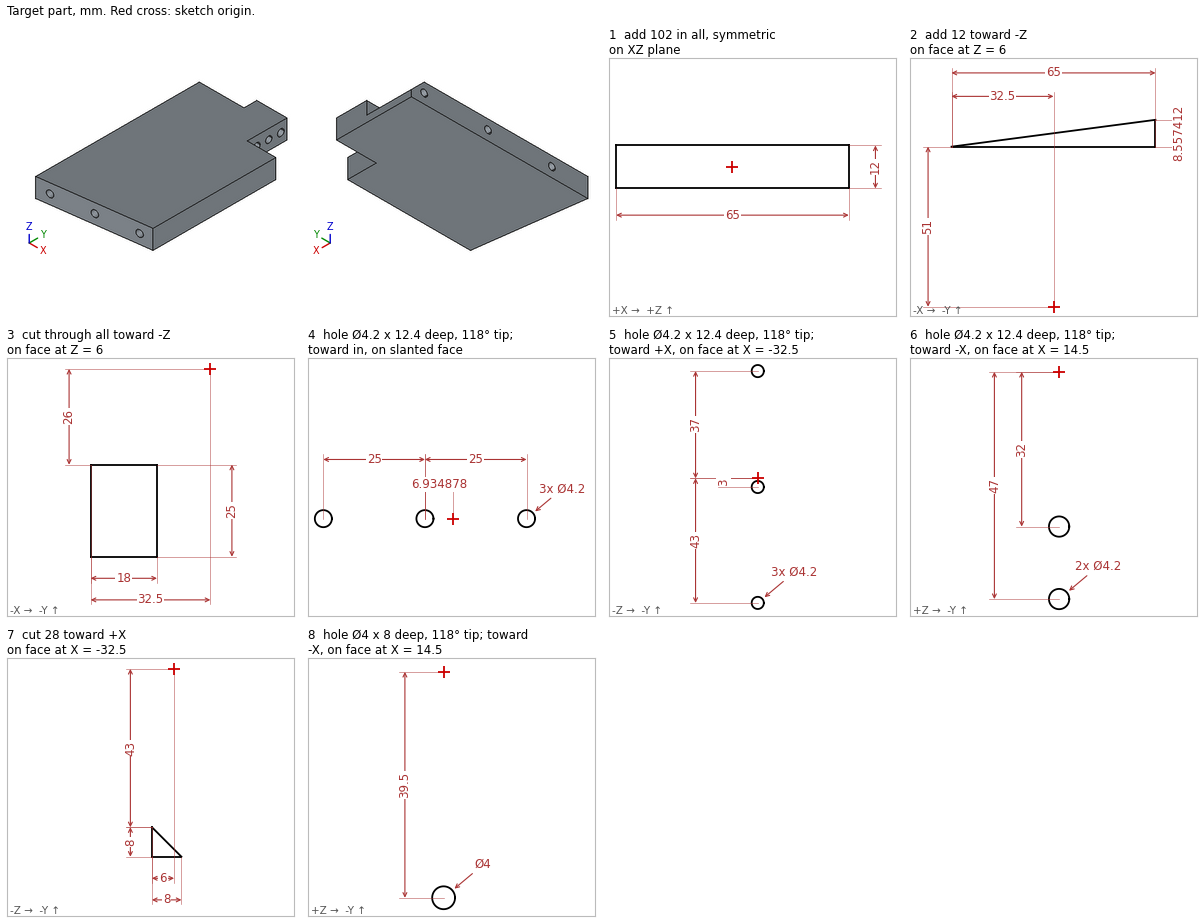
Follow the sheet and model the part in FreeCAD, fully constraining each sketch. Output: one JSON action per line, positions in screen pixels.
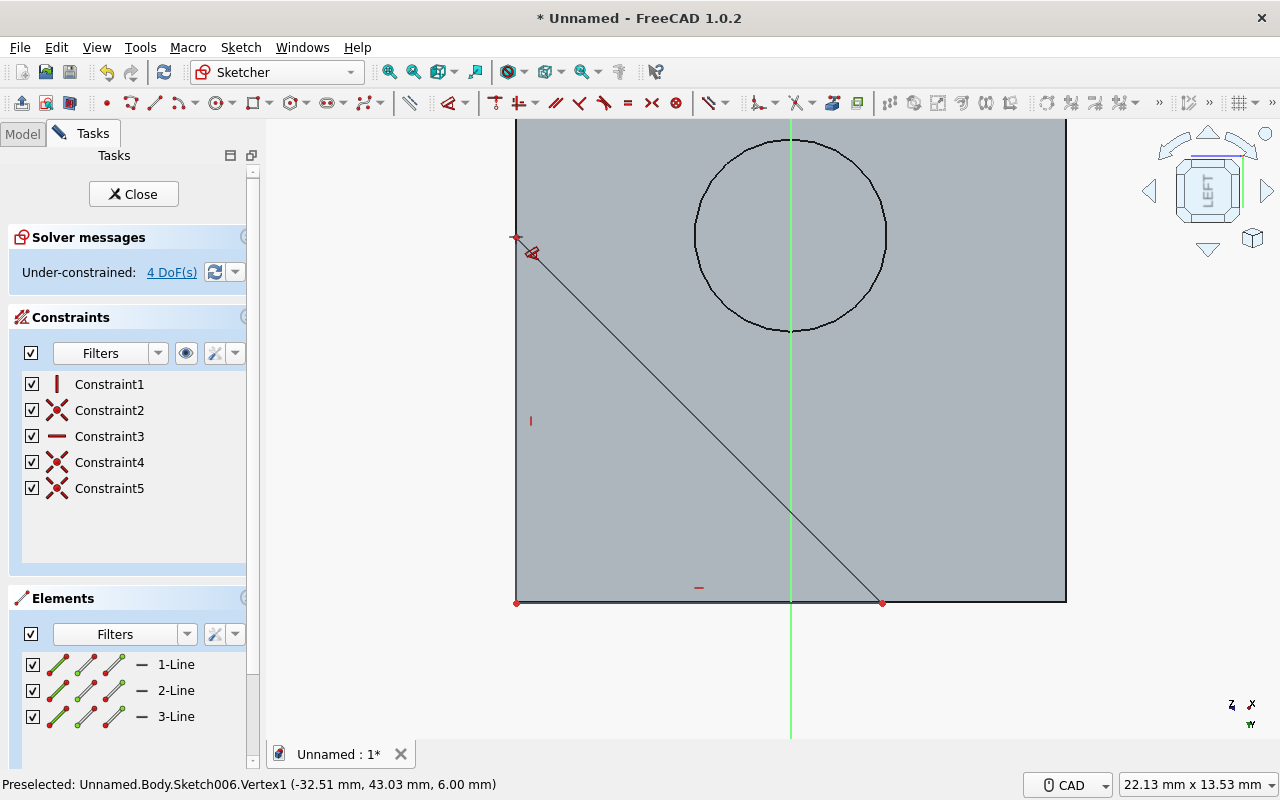
{"action": "left_click", "coordinate": [516, 347]}
{"action": "left_click", "coordinate": [482, 420]}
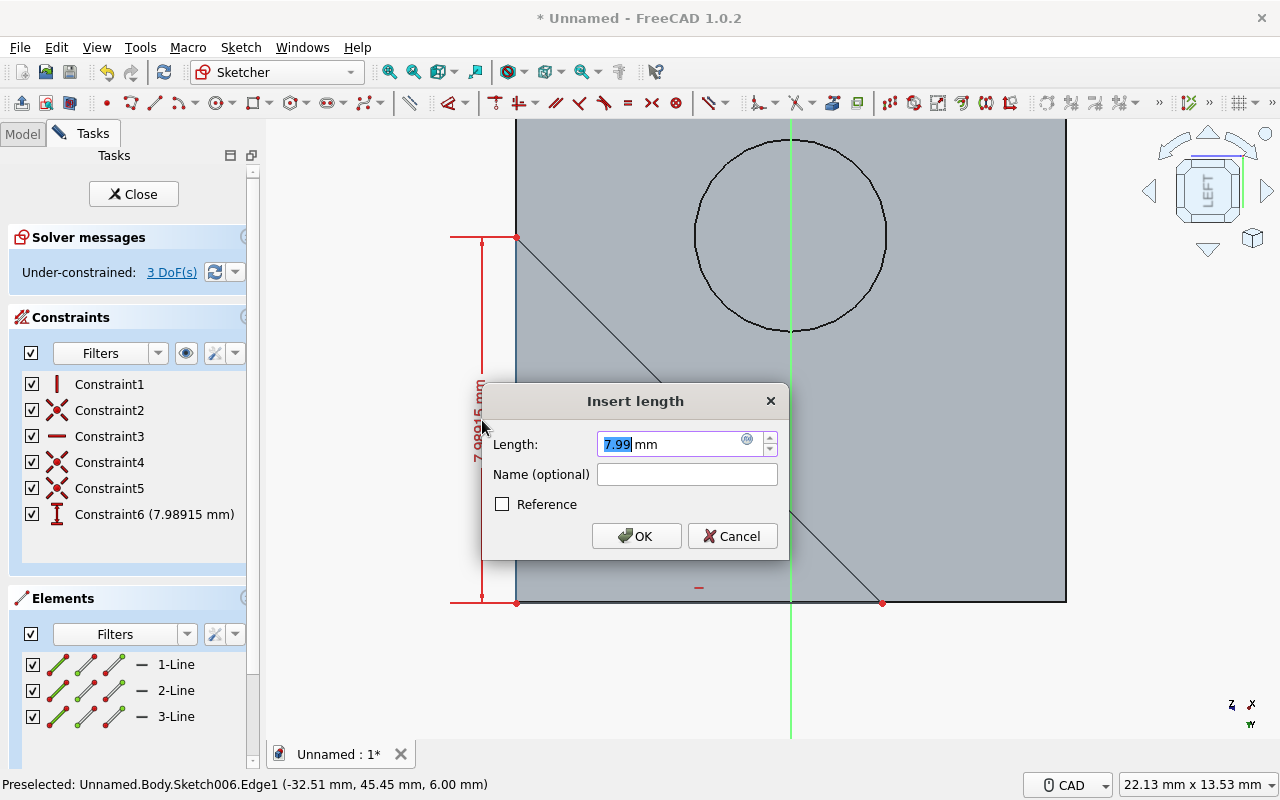
{"action": "type", "text": "8"}
{"action": "key", "text": "Return"}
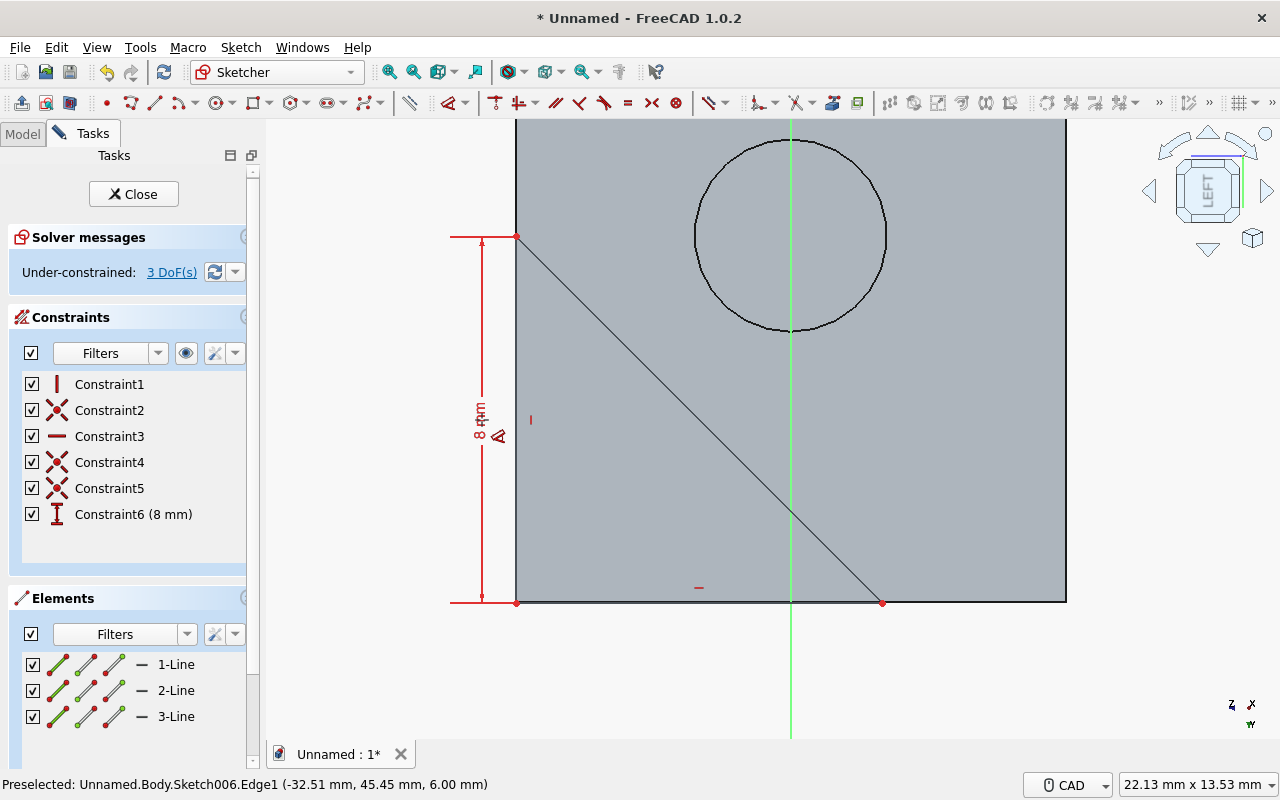
{"action": "left_click", "coordinate": [626, 603]}
{"action": "left_click", "coordinate": [699, 637]}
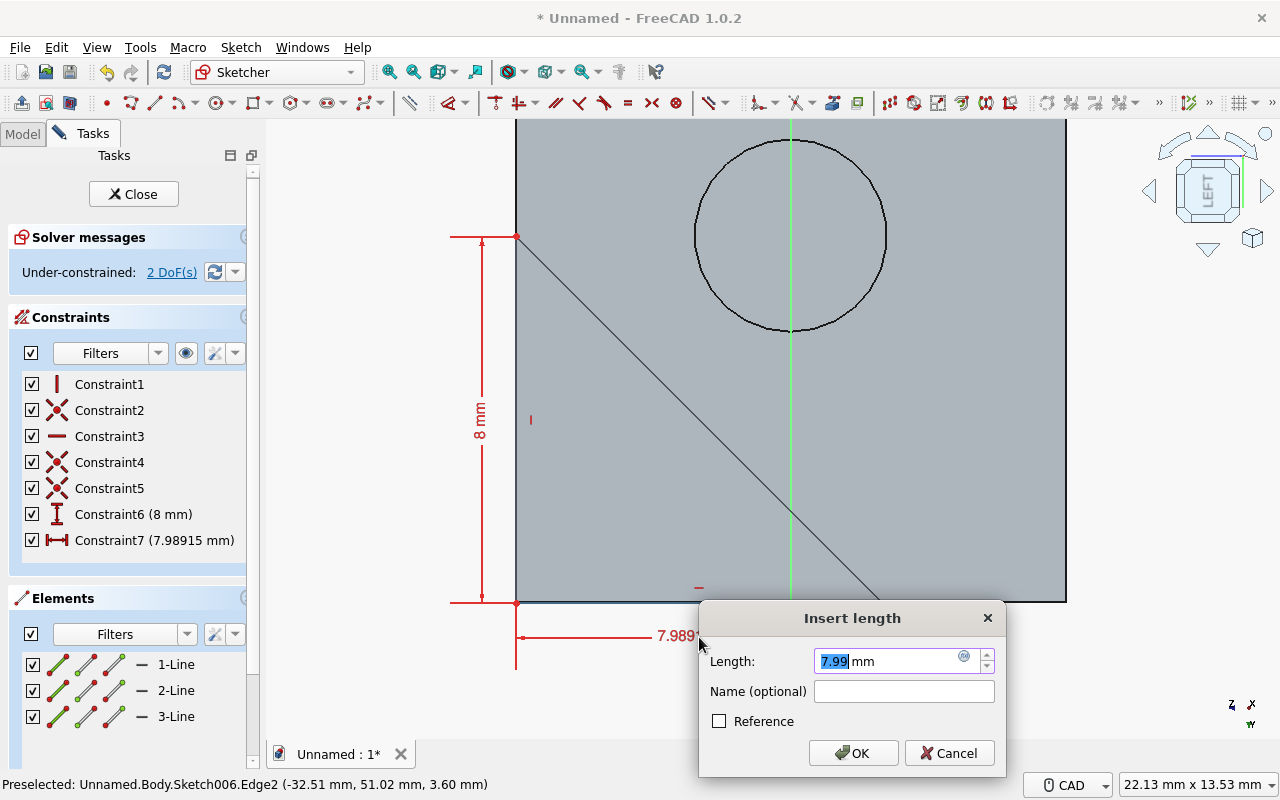
{"action": "type", "text": "8"}
{"action": "key", "text": "Return"}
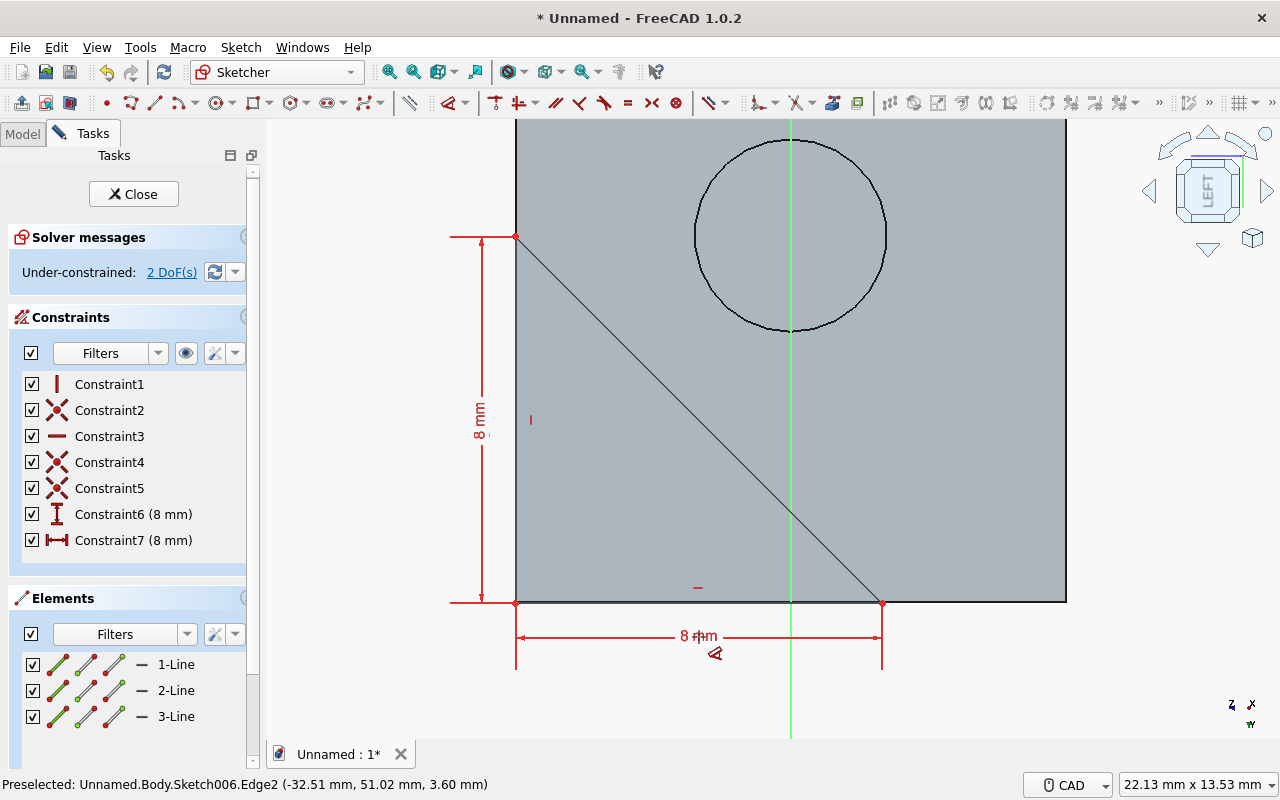
{"action": "left_click", "coordinate": [516, 237]}
{"action": "left_click", "coordinate": [653, 271]}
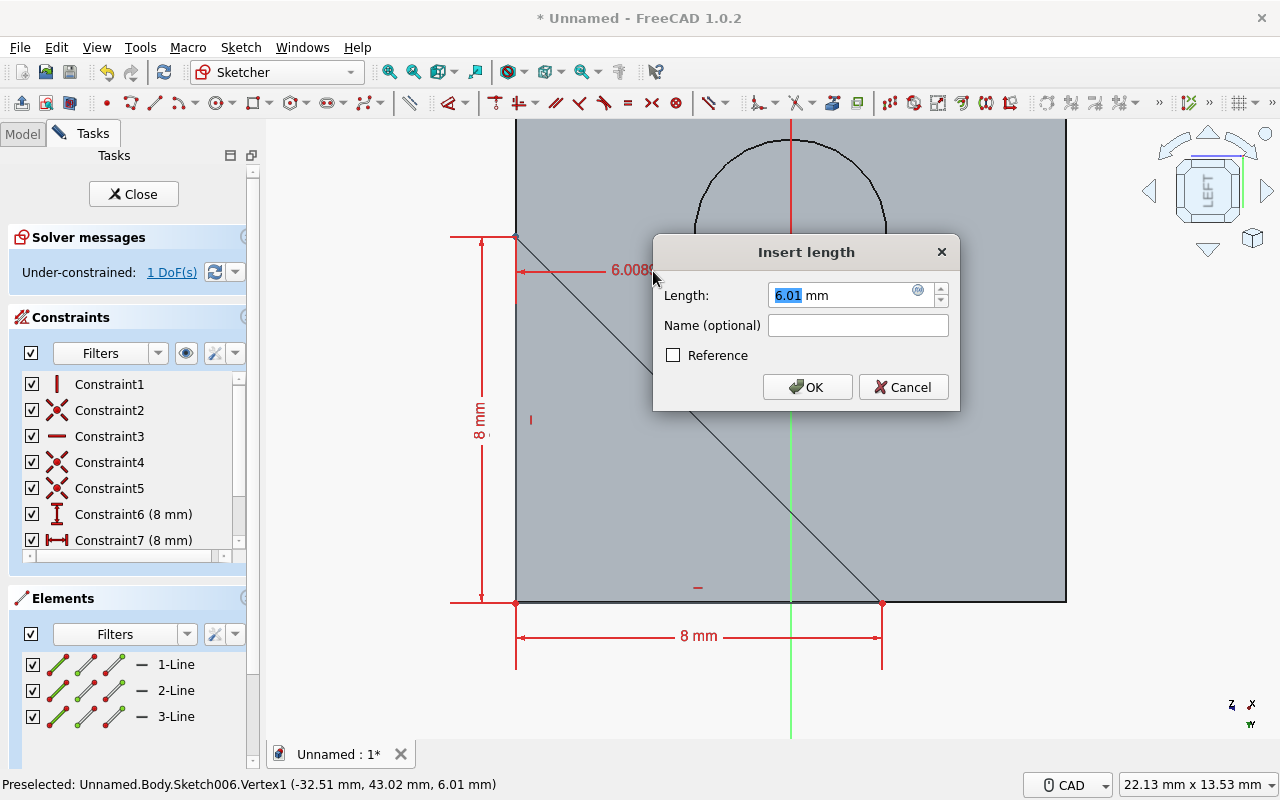
{"action": "type", "text": "6"}
{"action": "key", "text": "Return"}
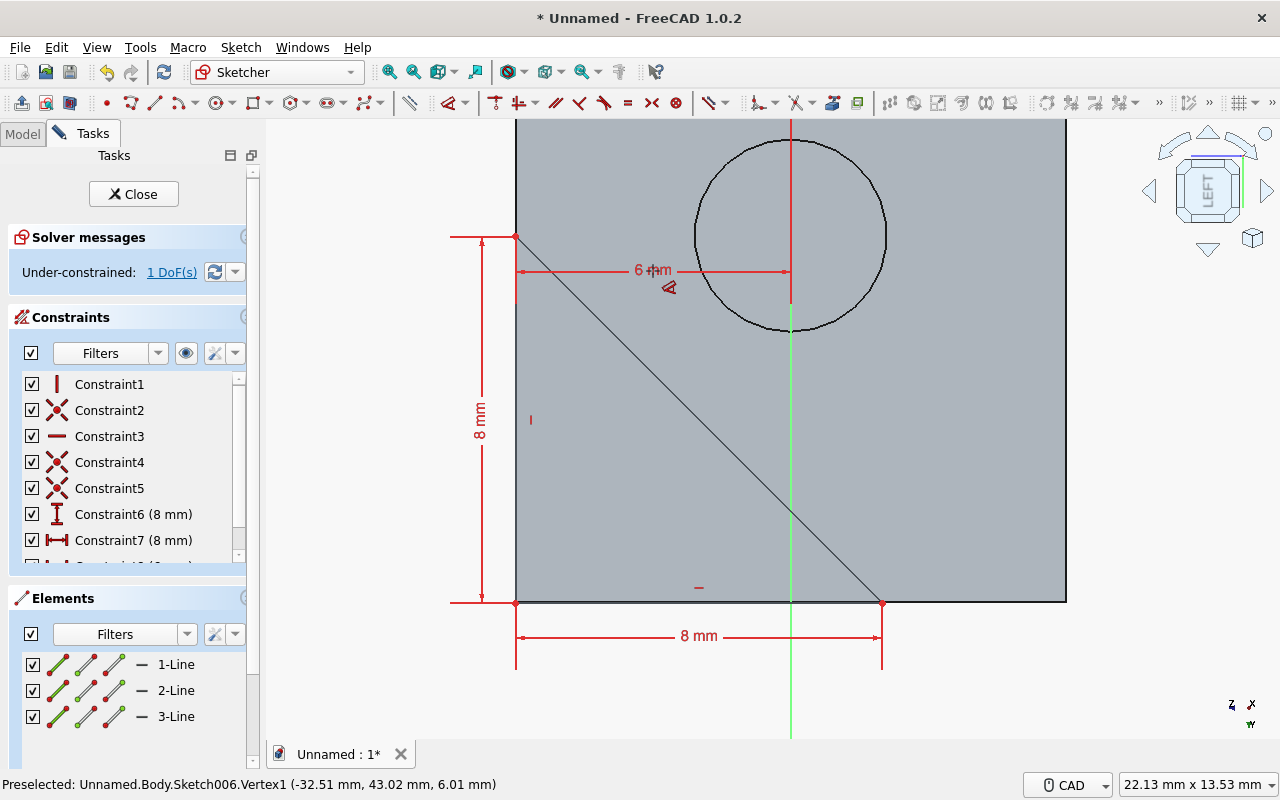
{"action": "left_click", "coordinate": [516, 237]}
{"action": "left_click", "coordinate": [482, 192]}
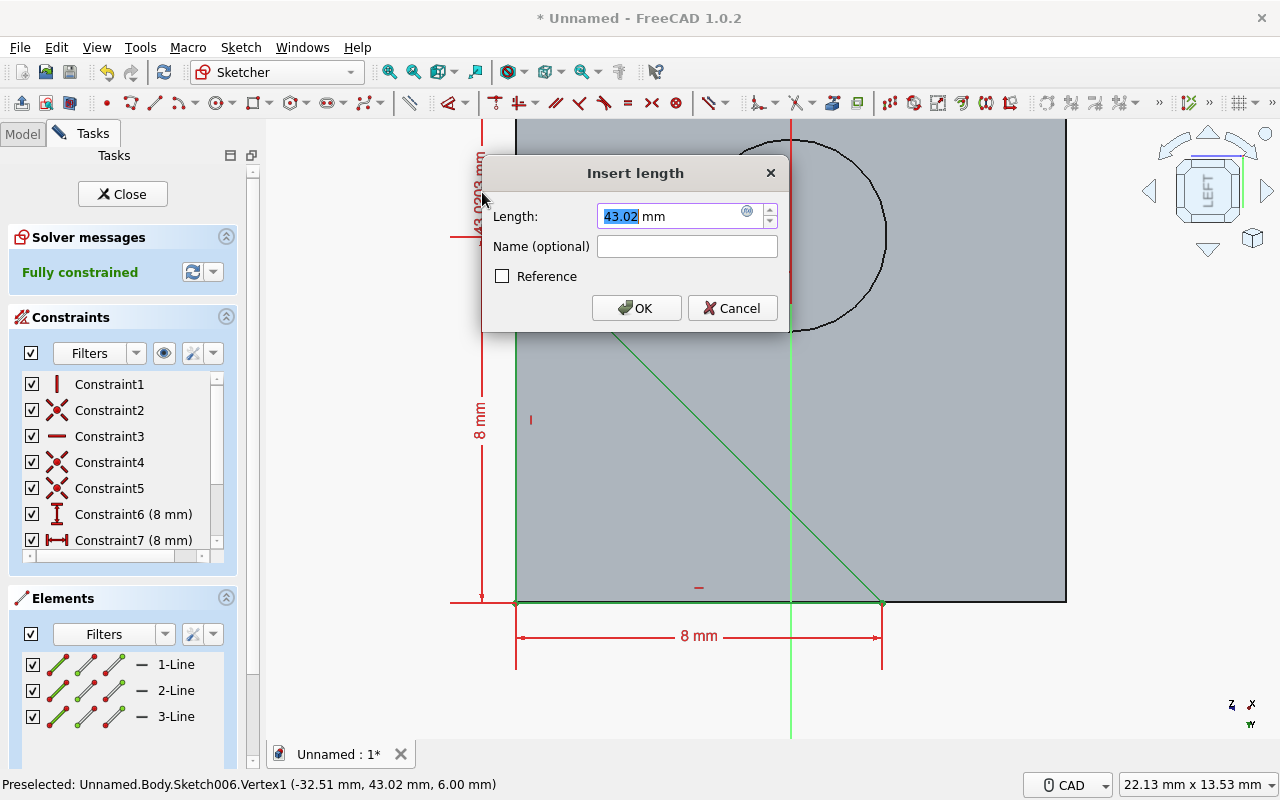
{"action": "type", "text": "43"}
{"action": "key", "text": "Return"}
{"action": "key", "text": "Escape"}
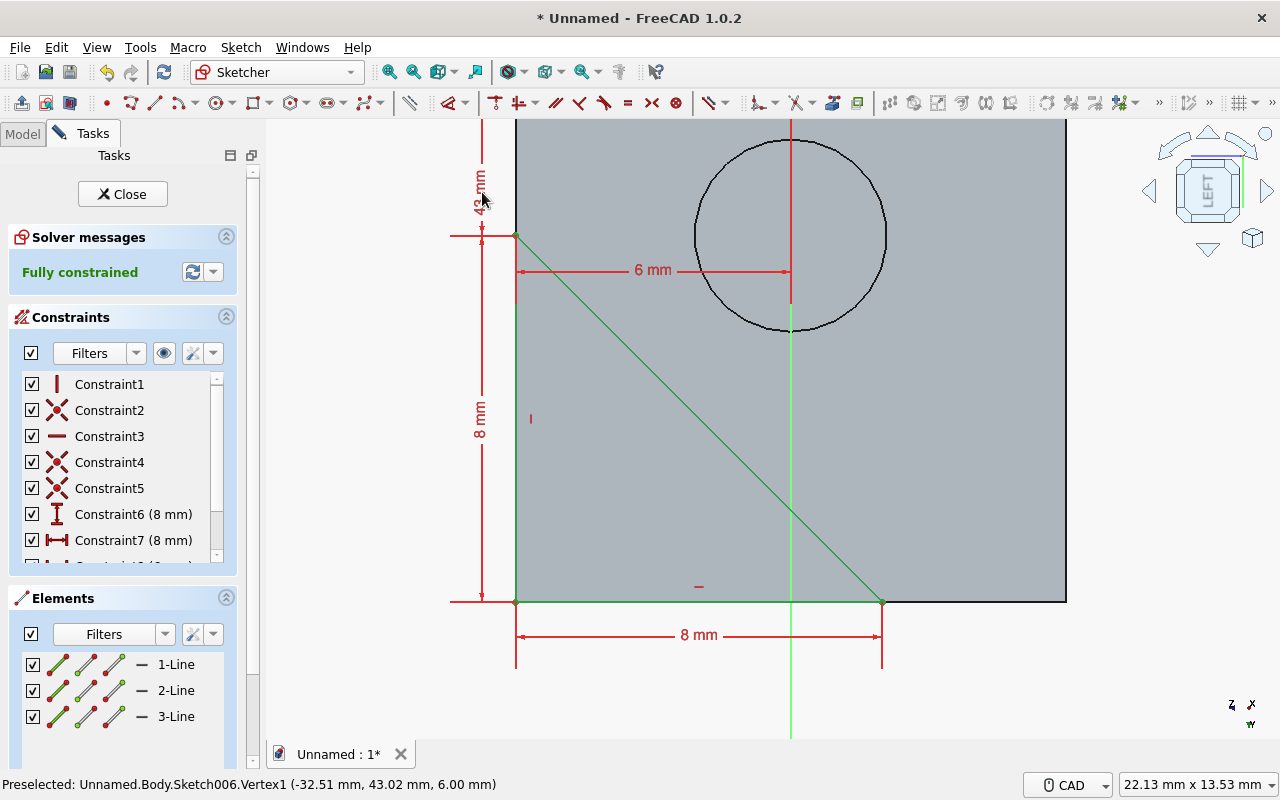
{"action": "left_click", "coordinate": [123, 194]}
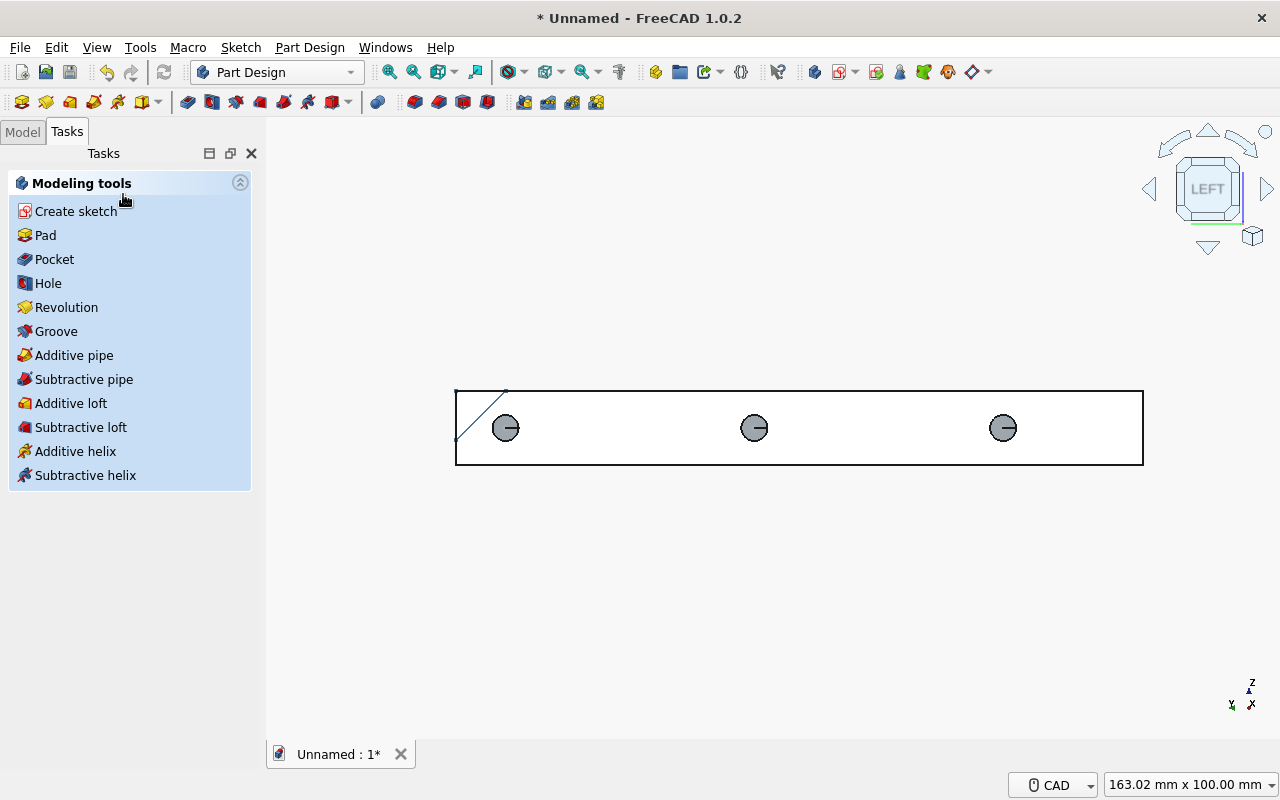
{"action": "left_click", "coordinate": [188, 102]}